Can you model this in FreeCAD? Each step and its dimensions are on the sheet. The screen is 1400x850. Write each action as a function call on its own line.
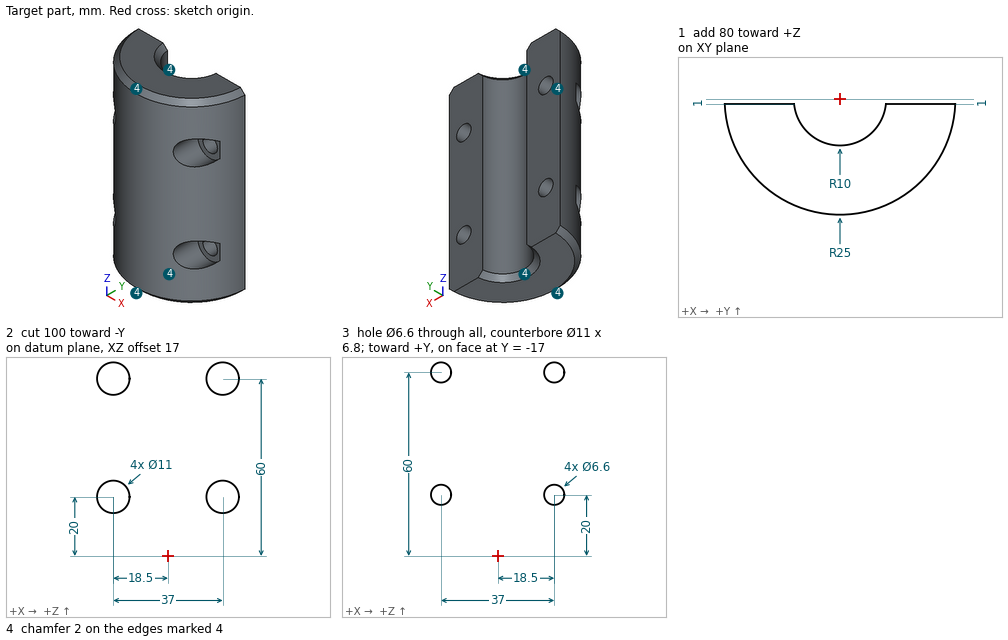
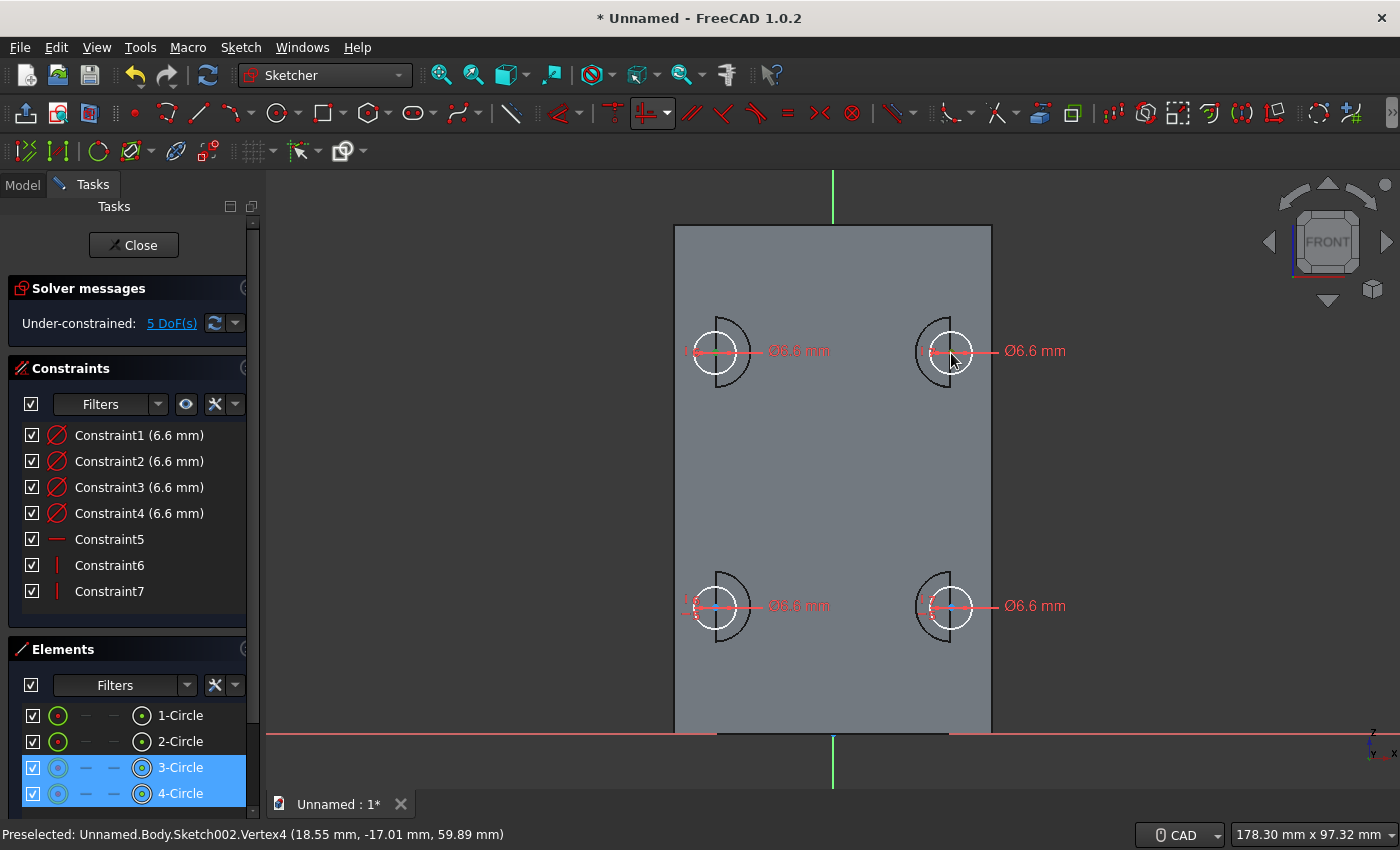
click(670, 114)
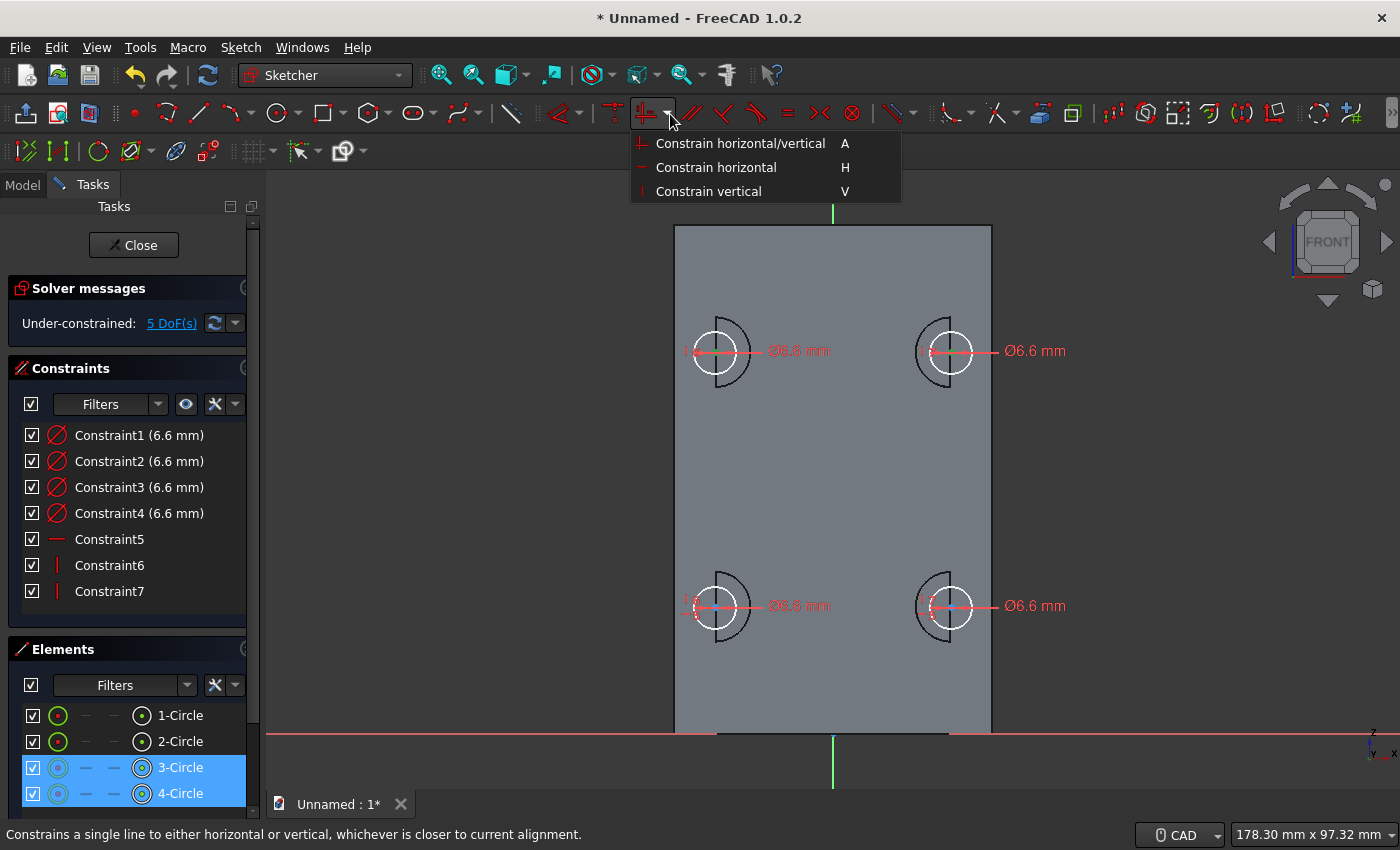
click(766, 167)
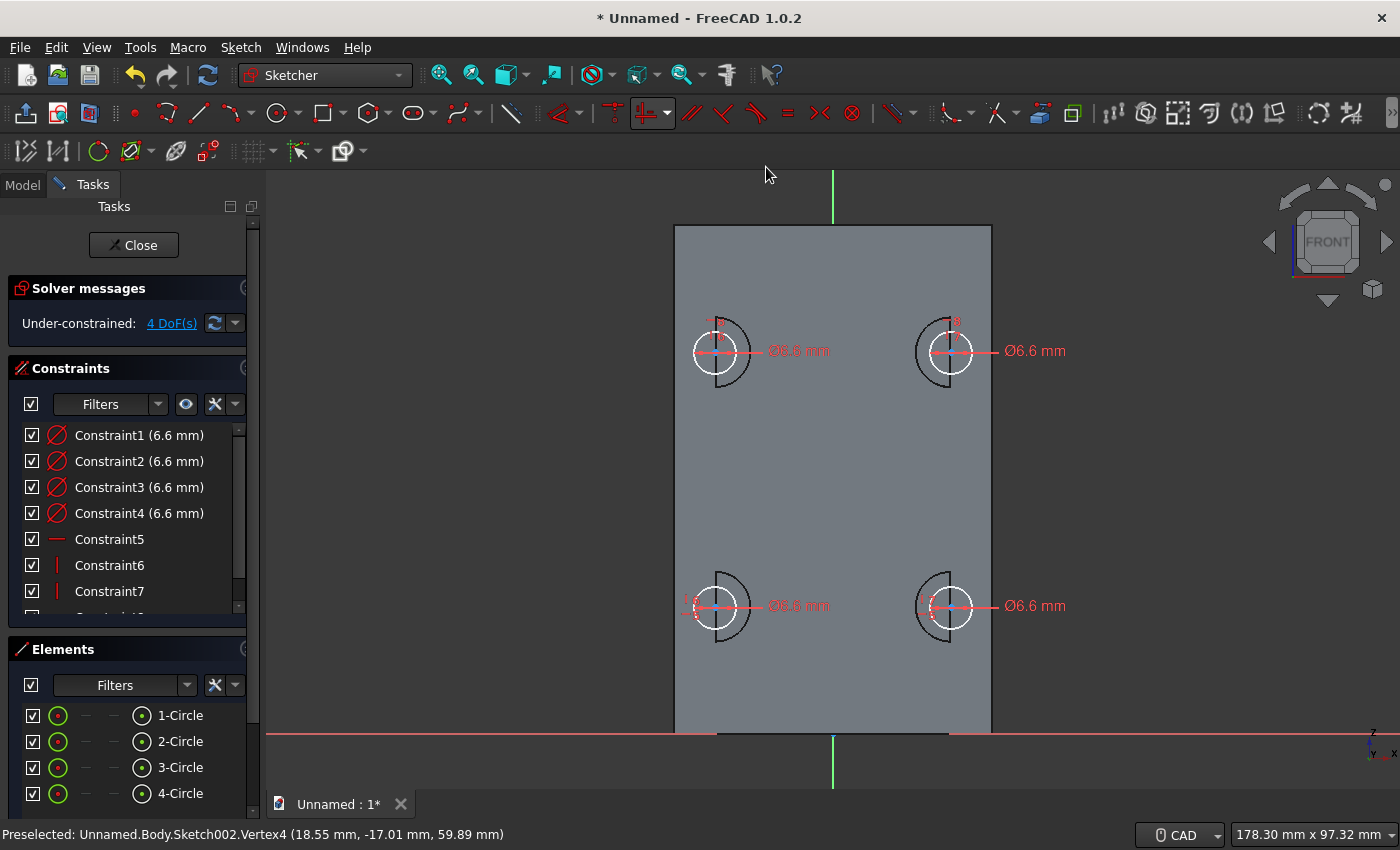
click(558, 114)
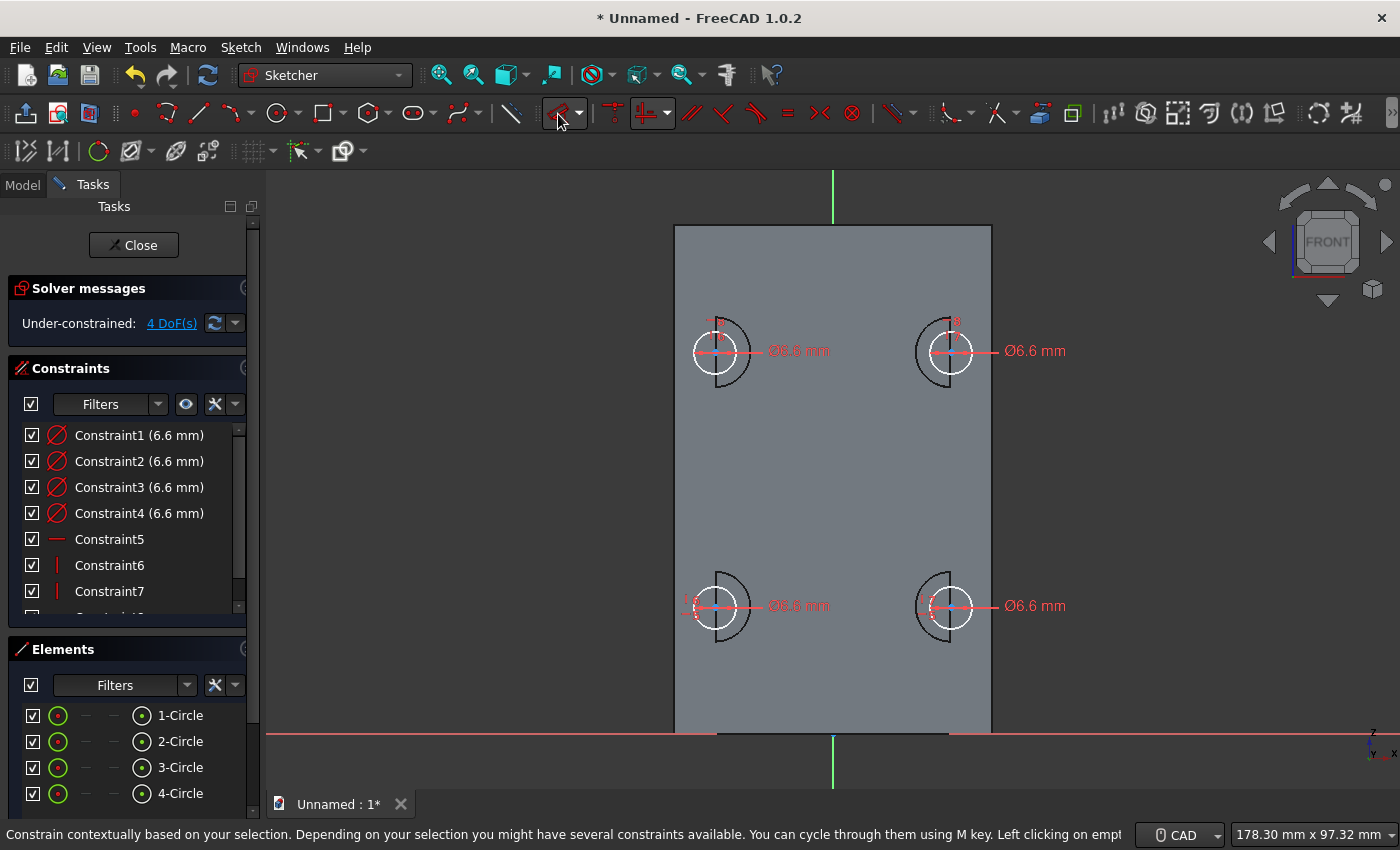
click(951, 608)
click(985, 671)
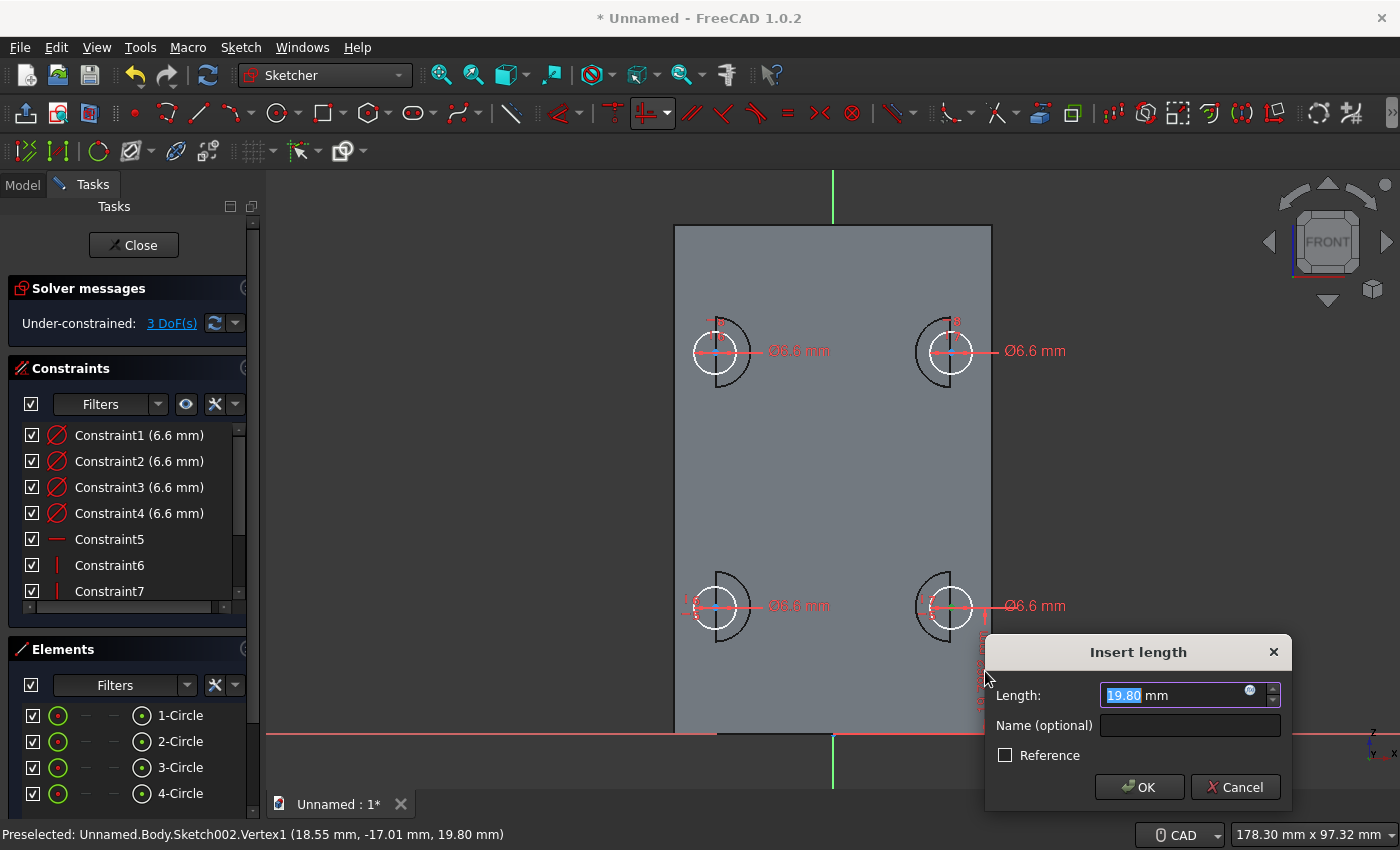
text(20)
key(Return)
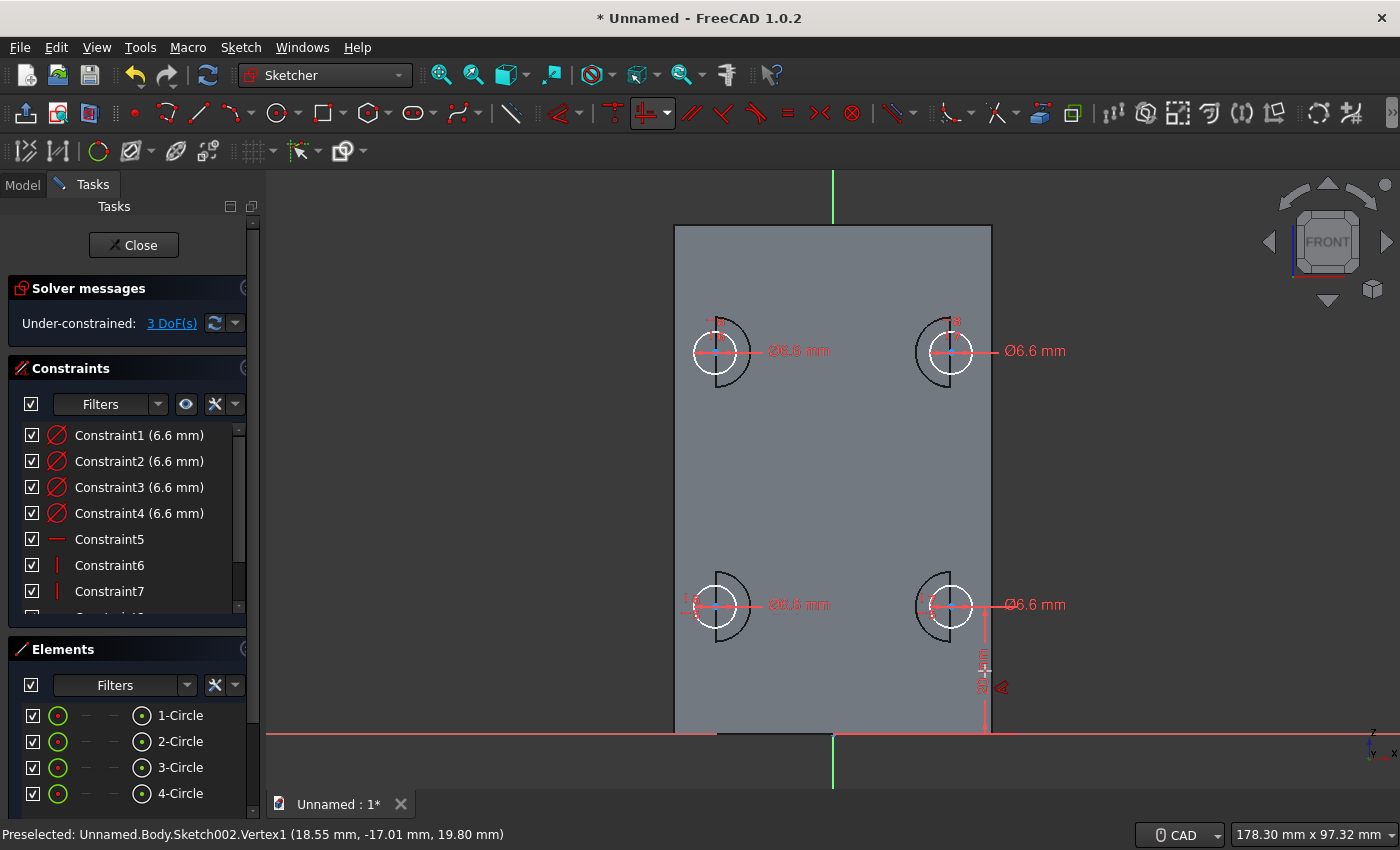
click(715, 353)
click(681, 543)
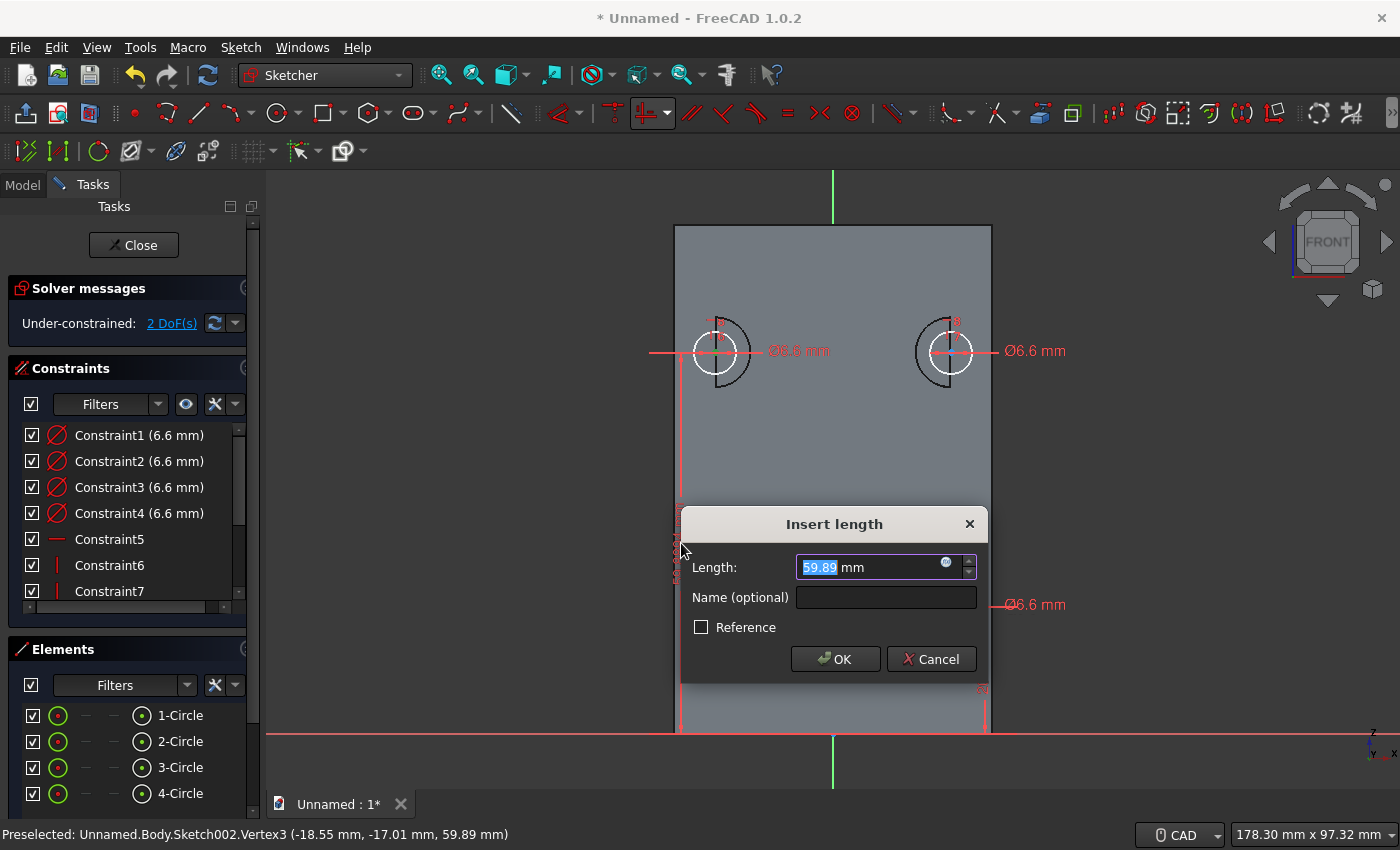
text(60)
key(Return)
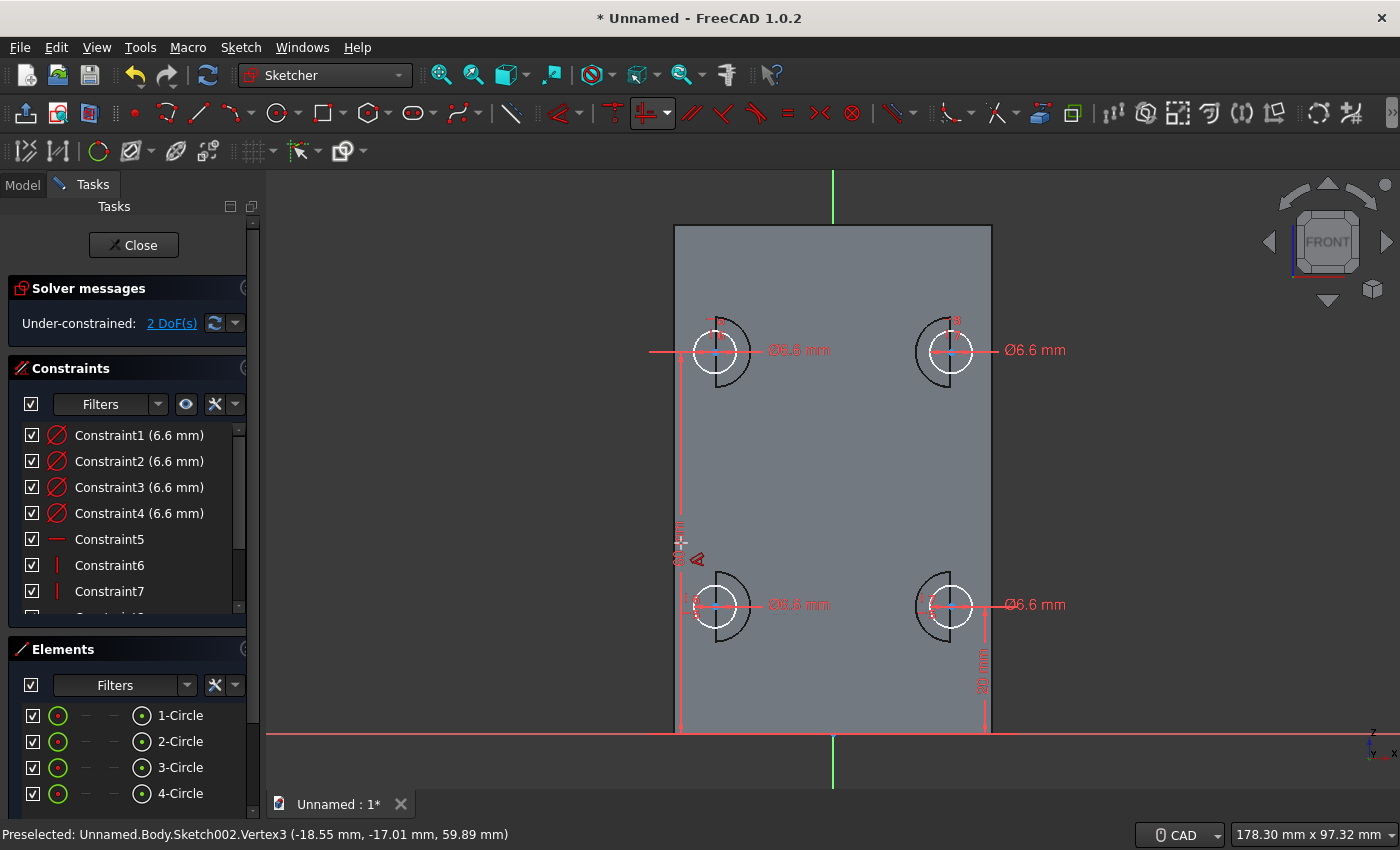
click(951, 607)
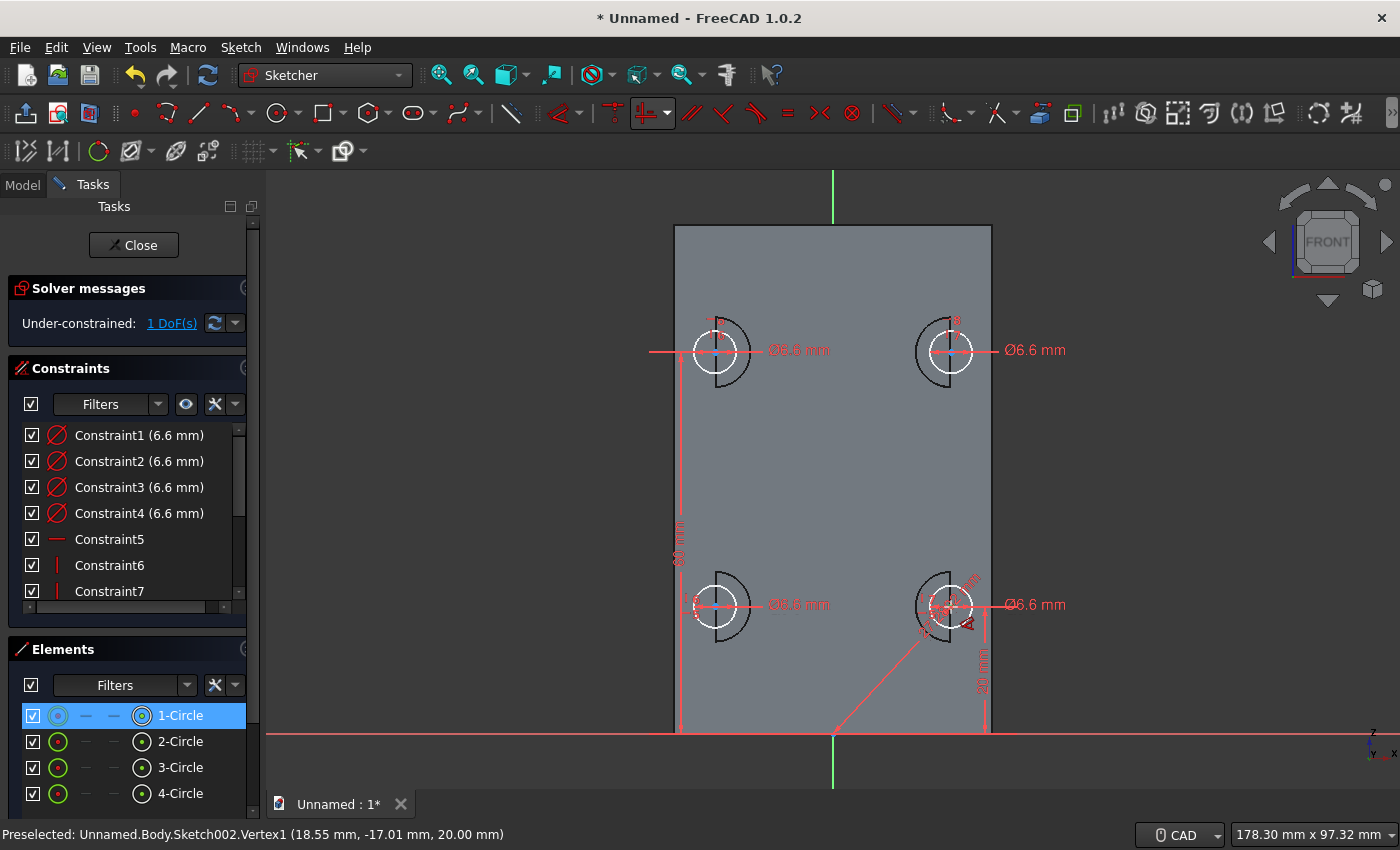
click(715, 607)
click(779, 641)